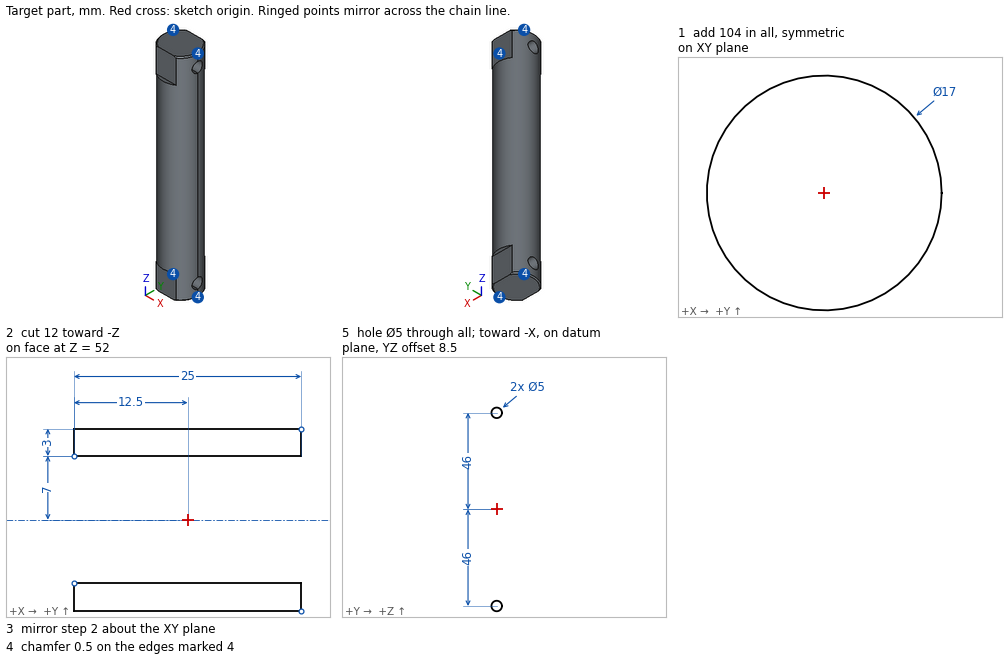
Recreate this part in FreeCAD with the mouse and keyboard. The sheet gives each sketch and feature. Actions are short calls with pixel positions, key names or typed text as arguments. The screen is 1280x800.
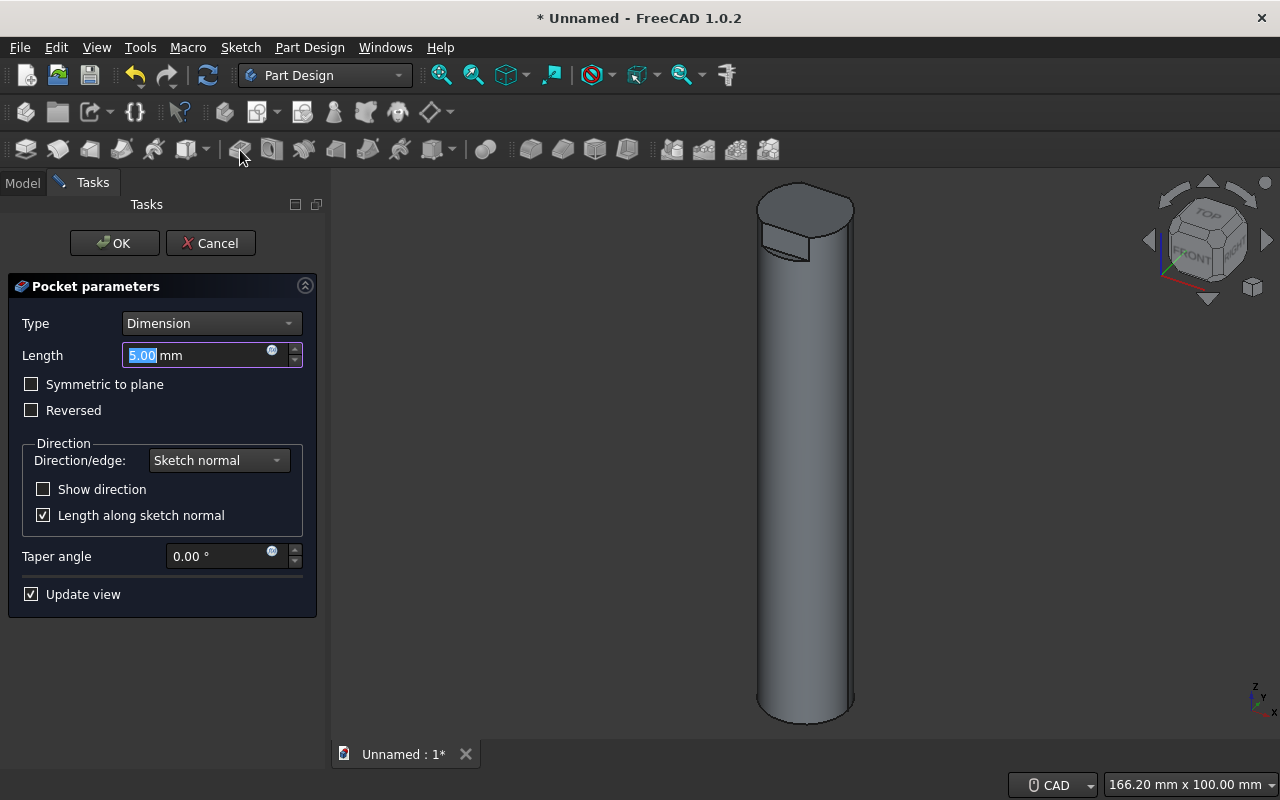
text(12)
key(Tab)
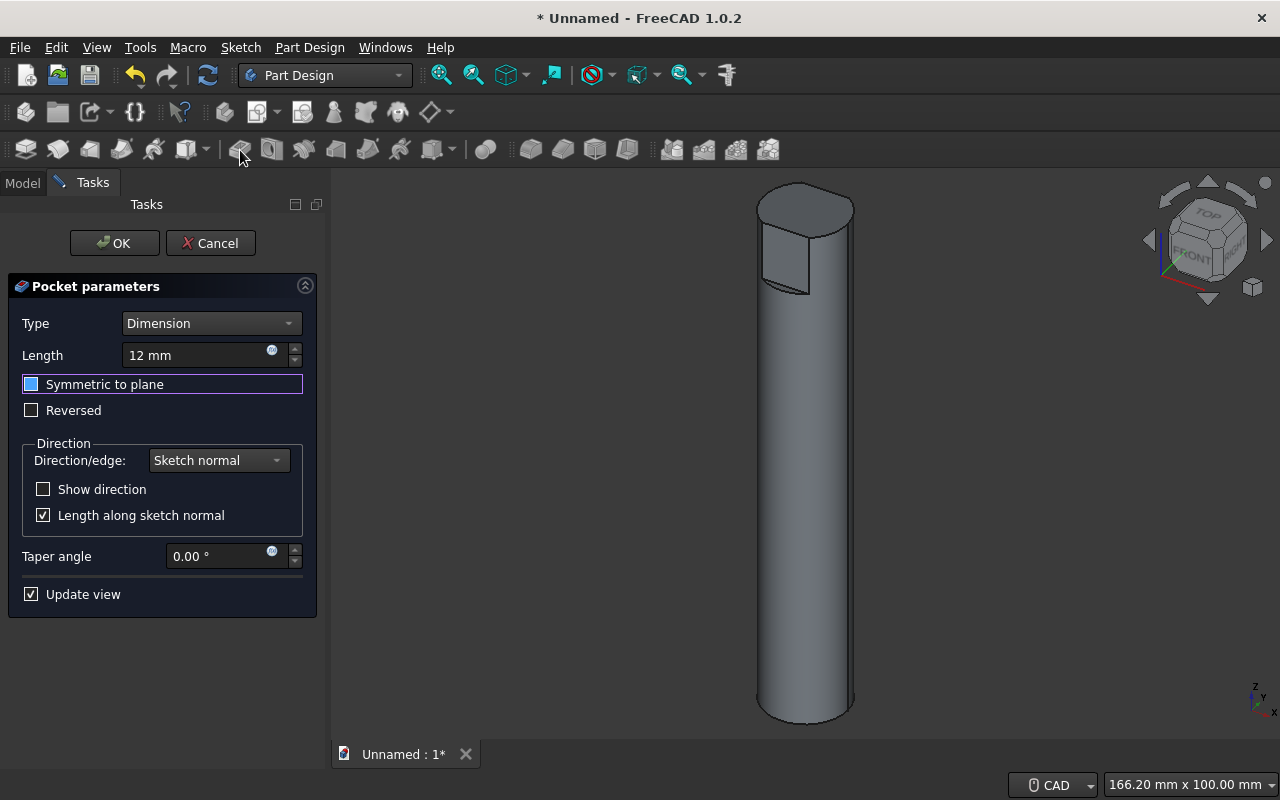
click(115, 243)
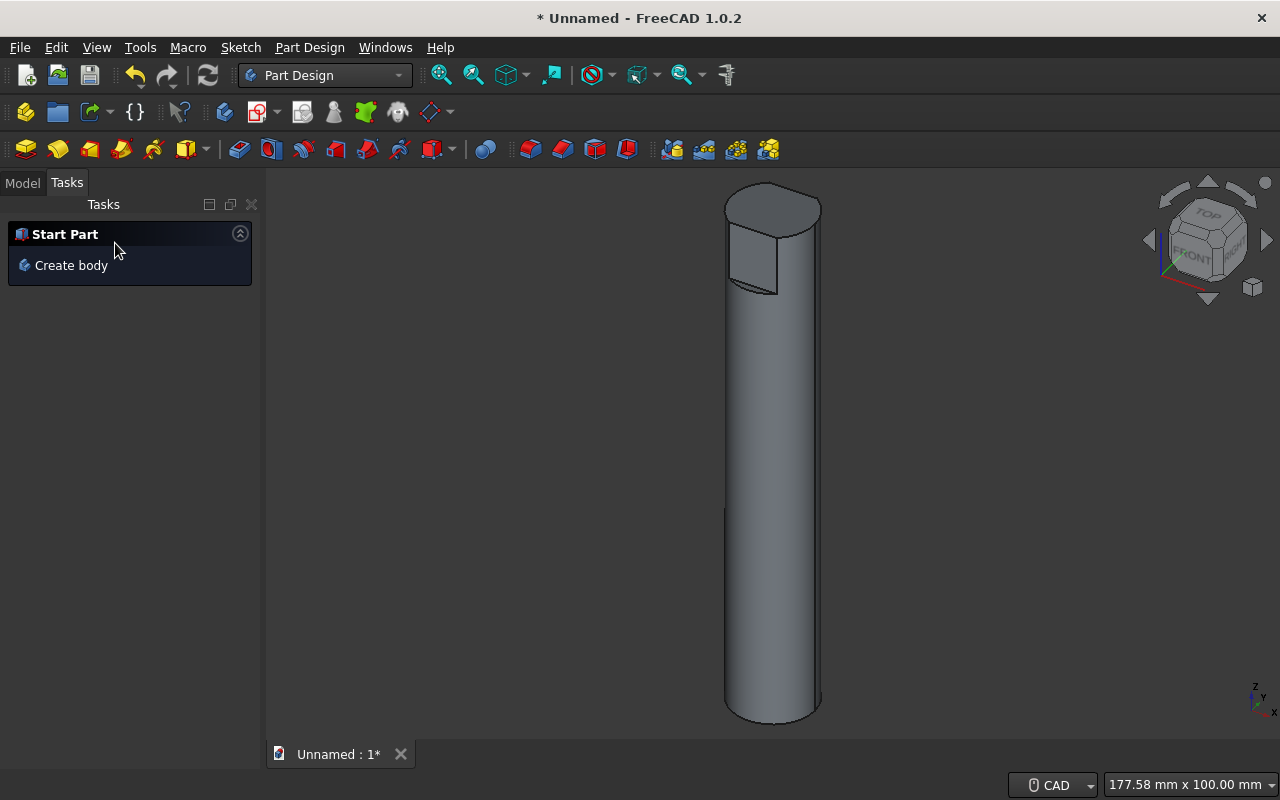
click(23, 182)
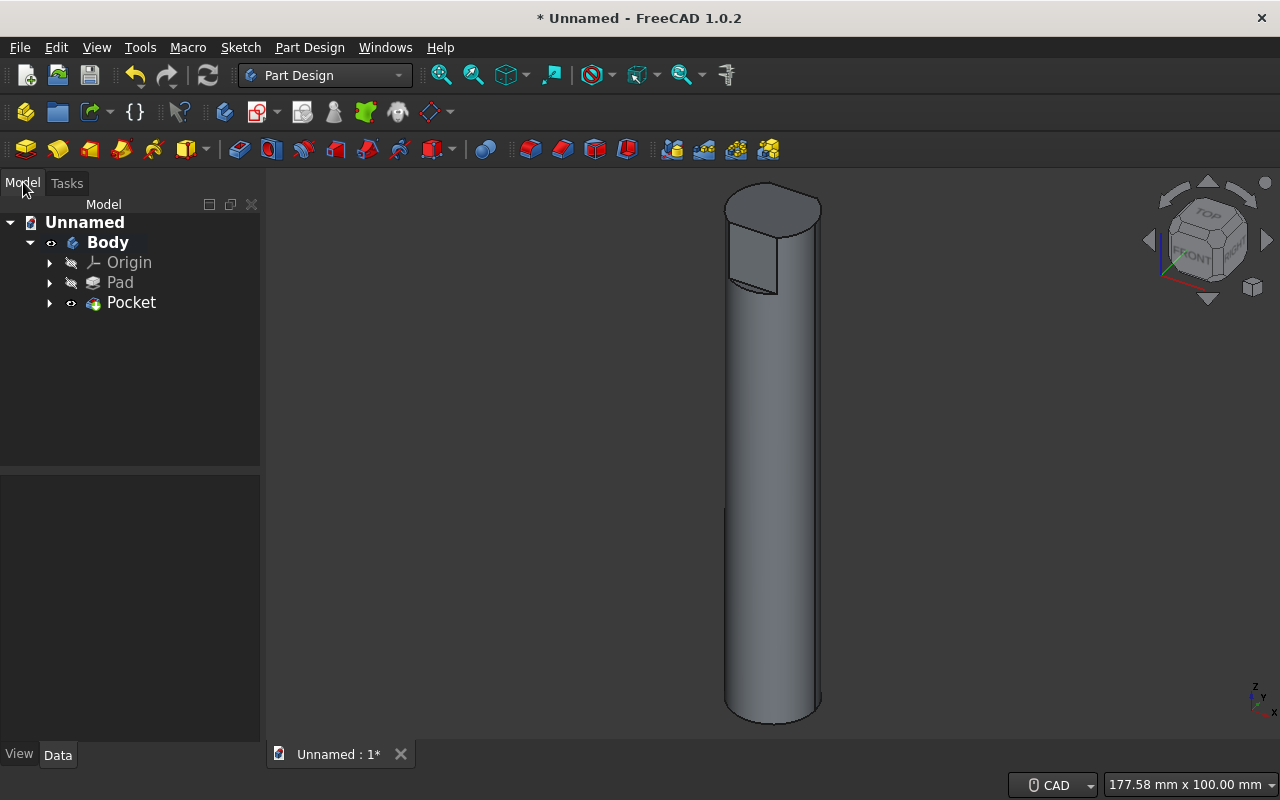
click(116, 303)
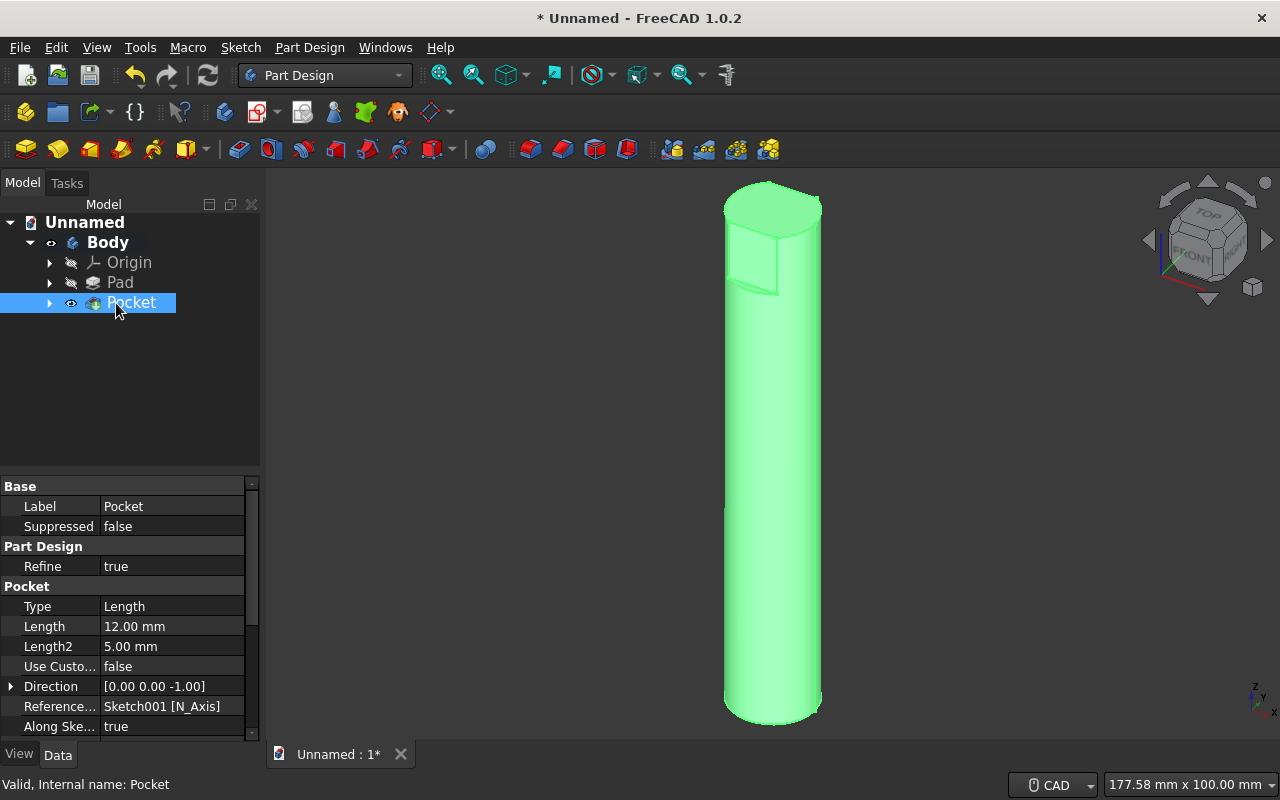
click(672, 150)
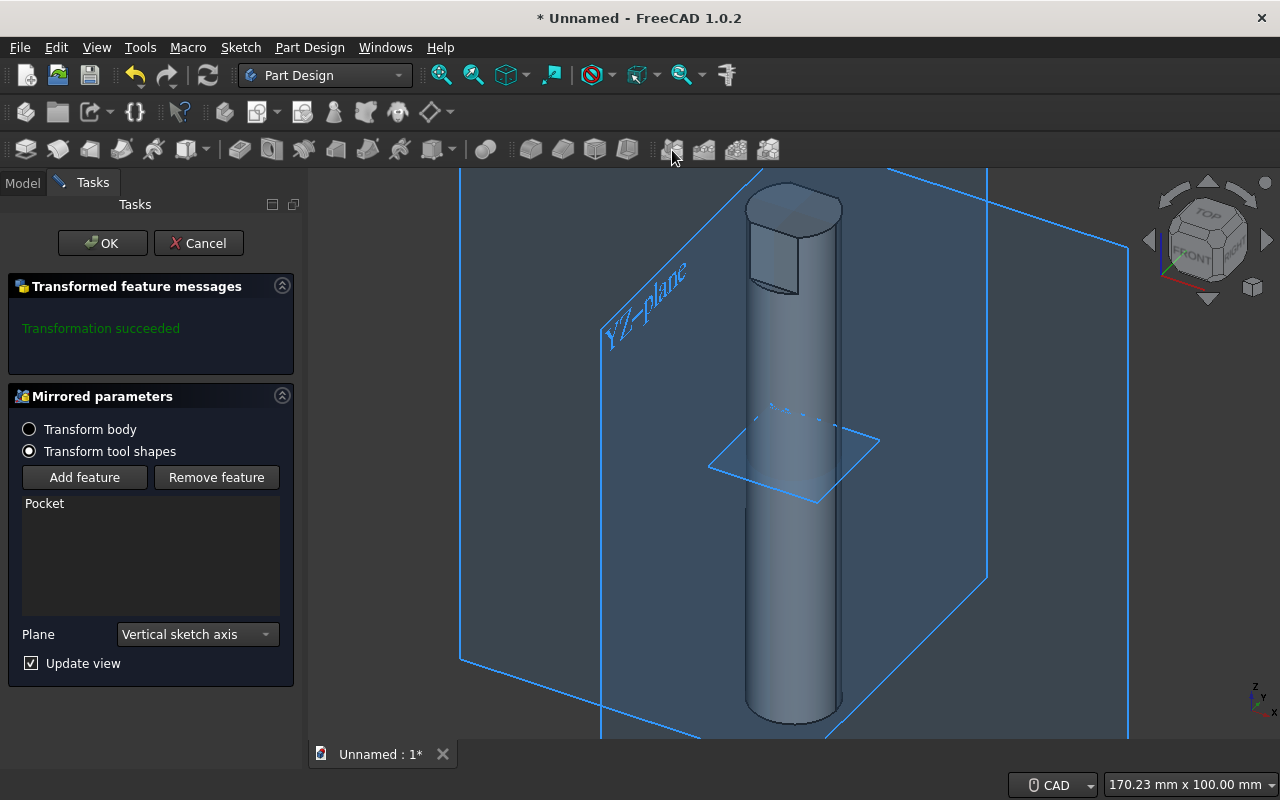
click(198, 634)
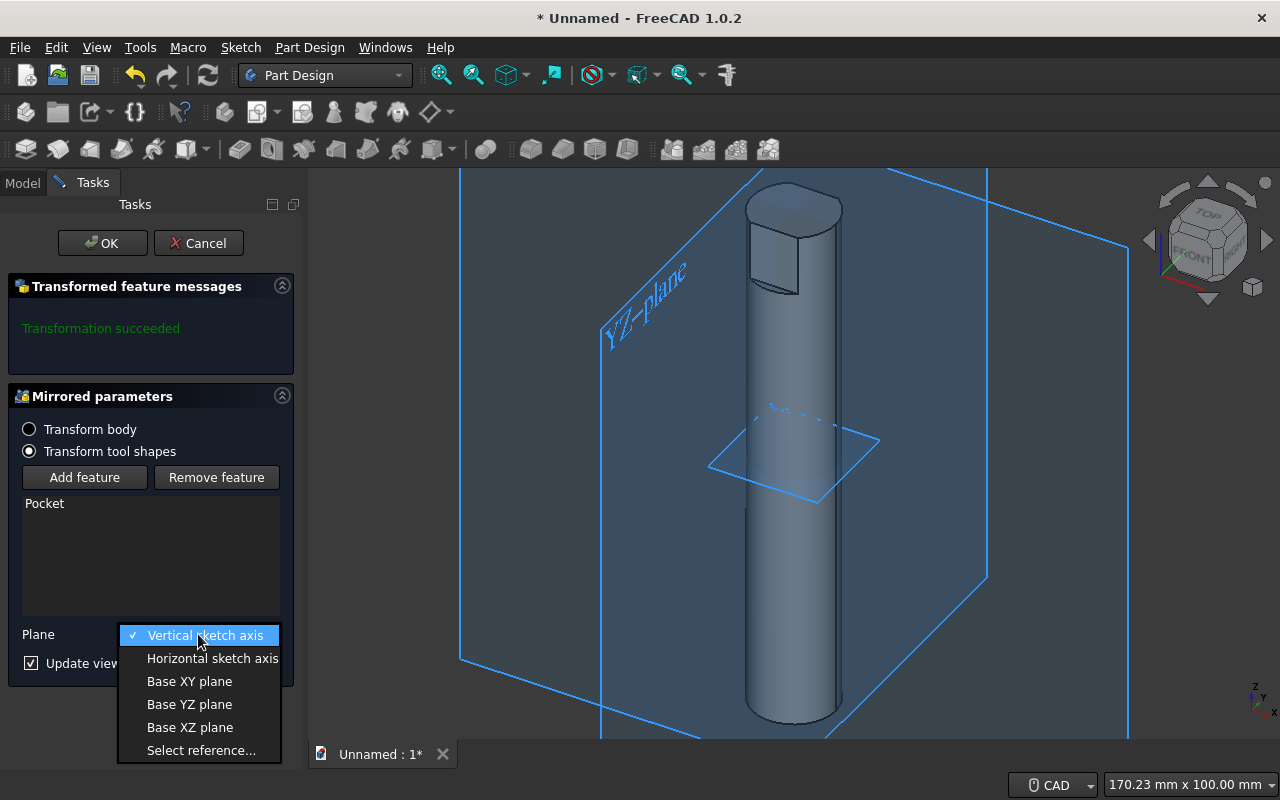
click(198, 682)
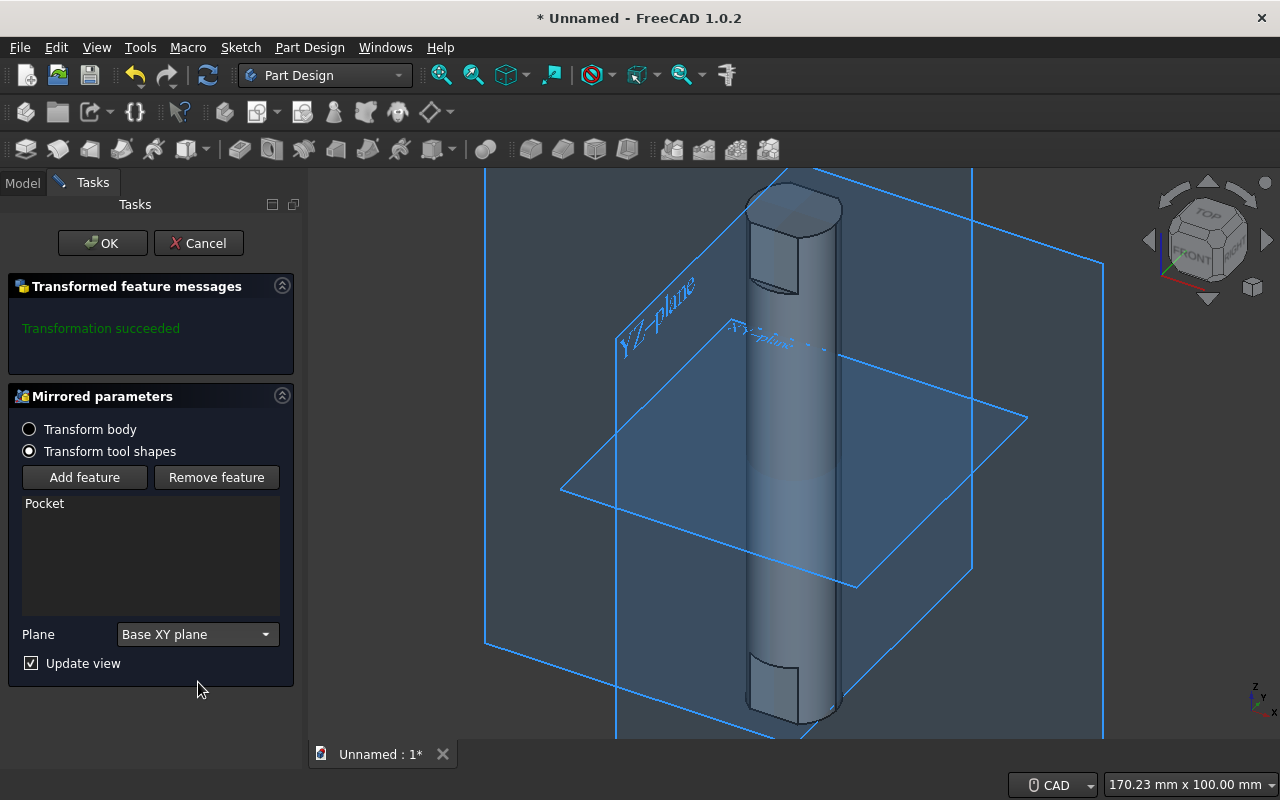
click(103, 243)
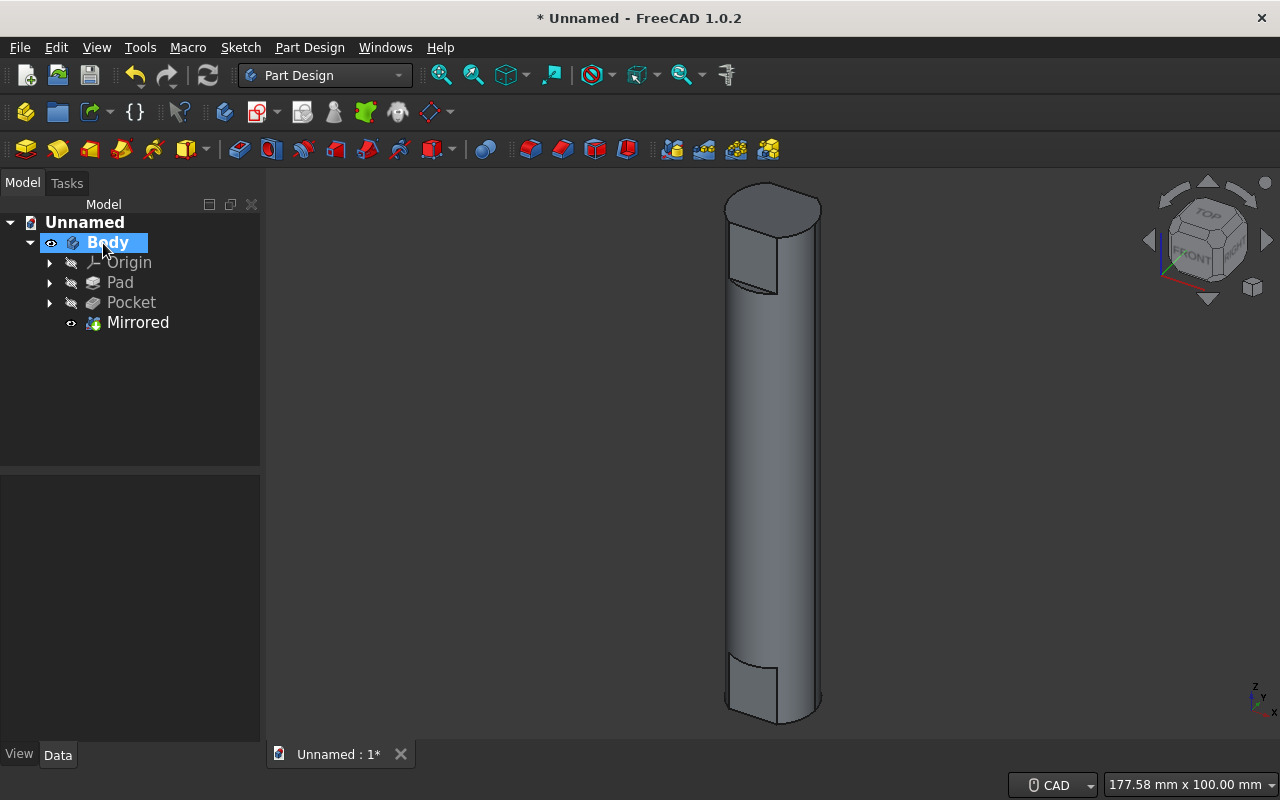
click(799, 233)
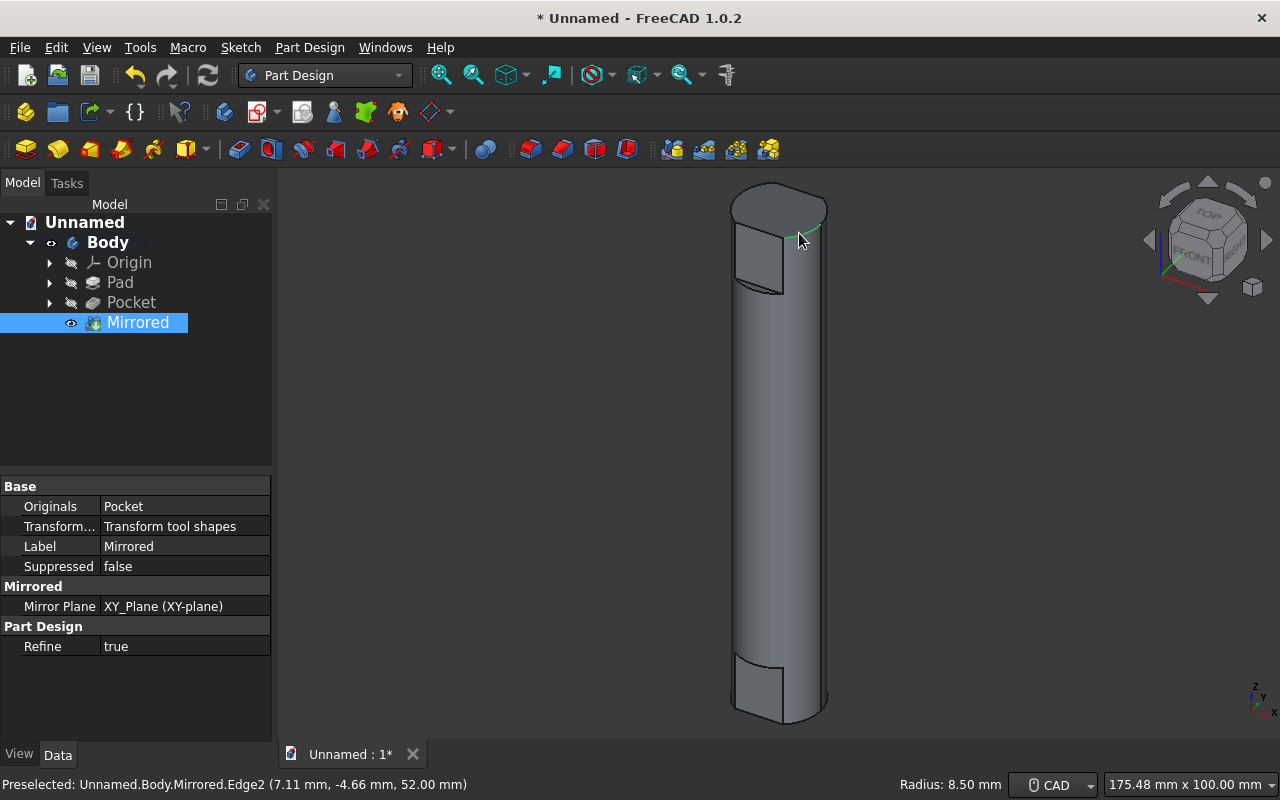
click(731, 211, ctrl)